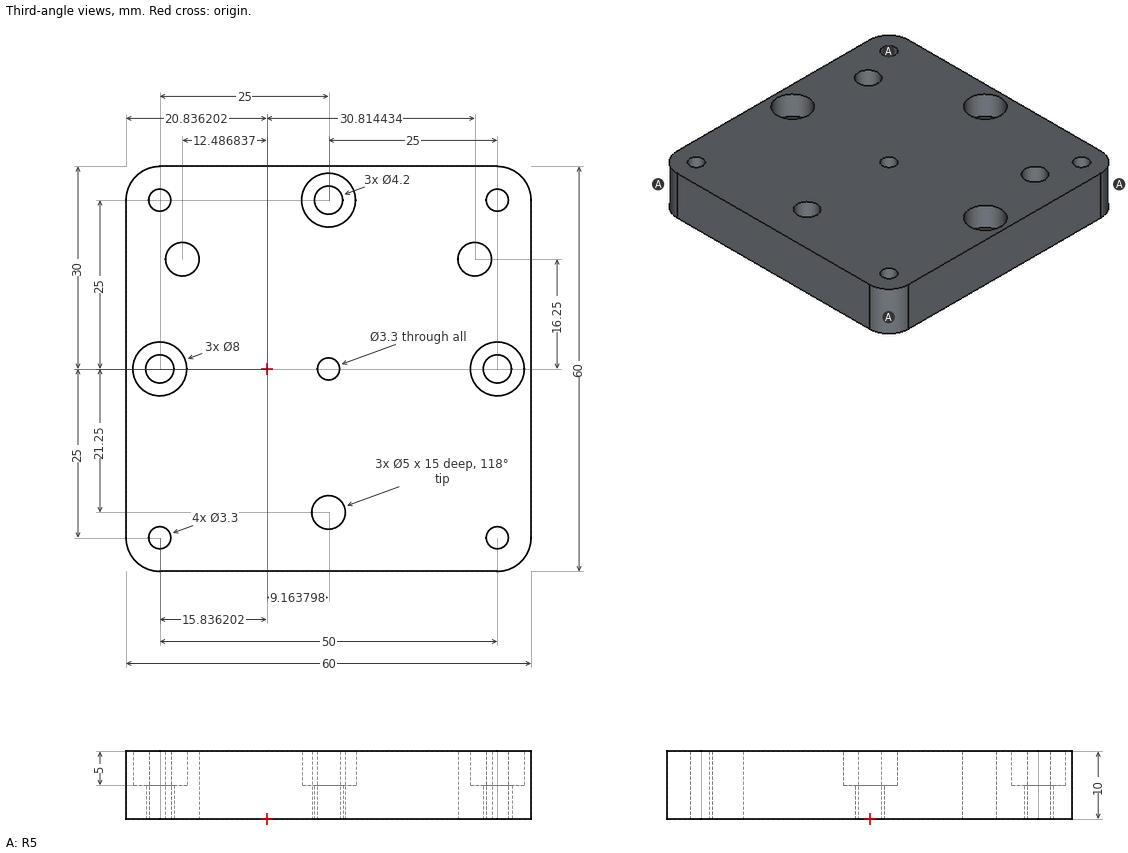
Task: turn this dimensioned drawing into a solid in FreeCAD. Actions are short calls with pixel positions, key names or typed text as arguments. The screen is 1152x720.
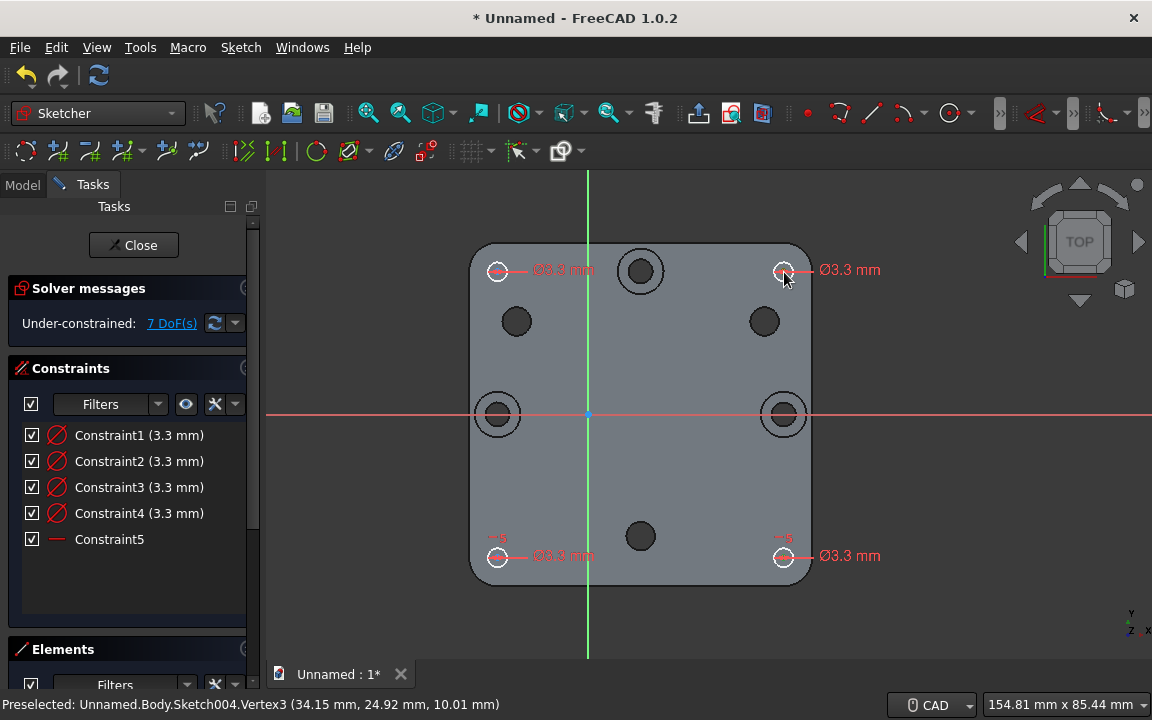
key(v)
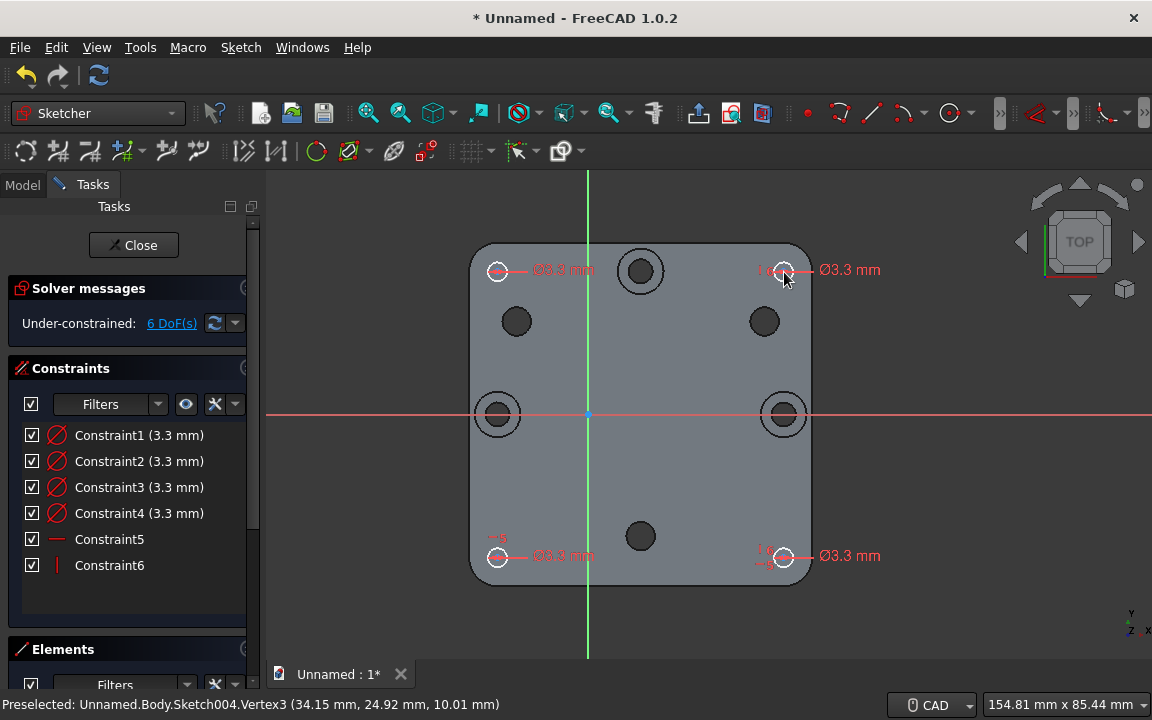
click(498, 558)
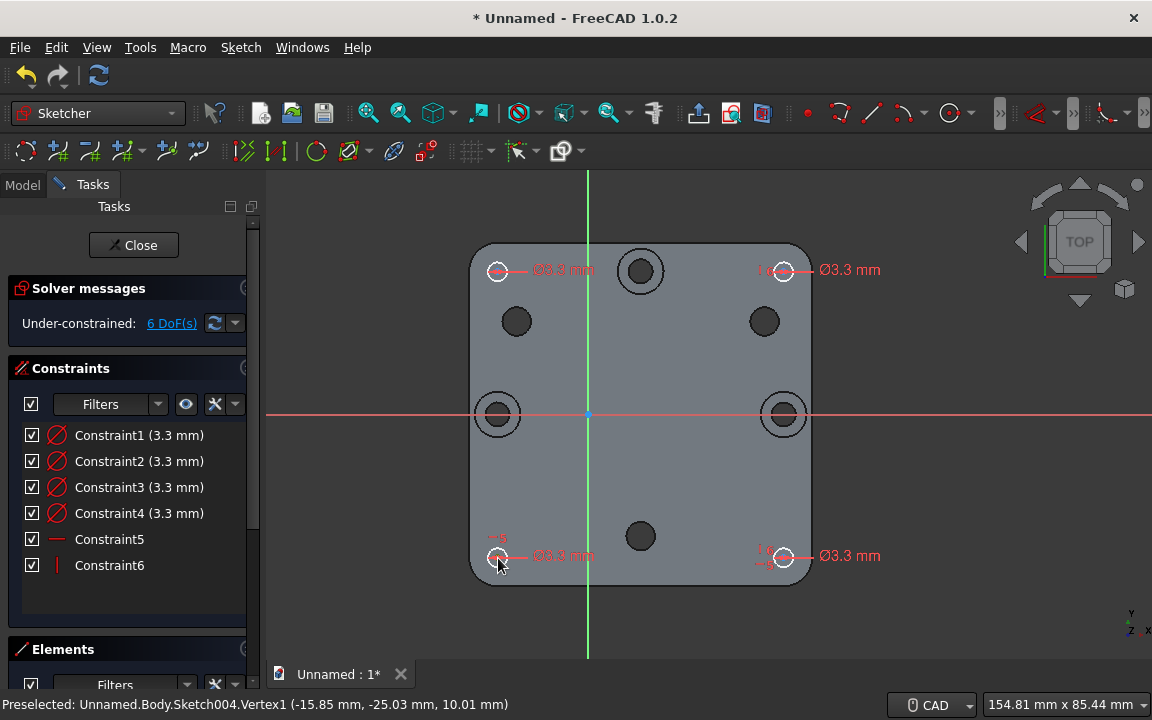
click(497, 272)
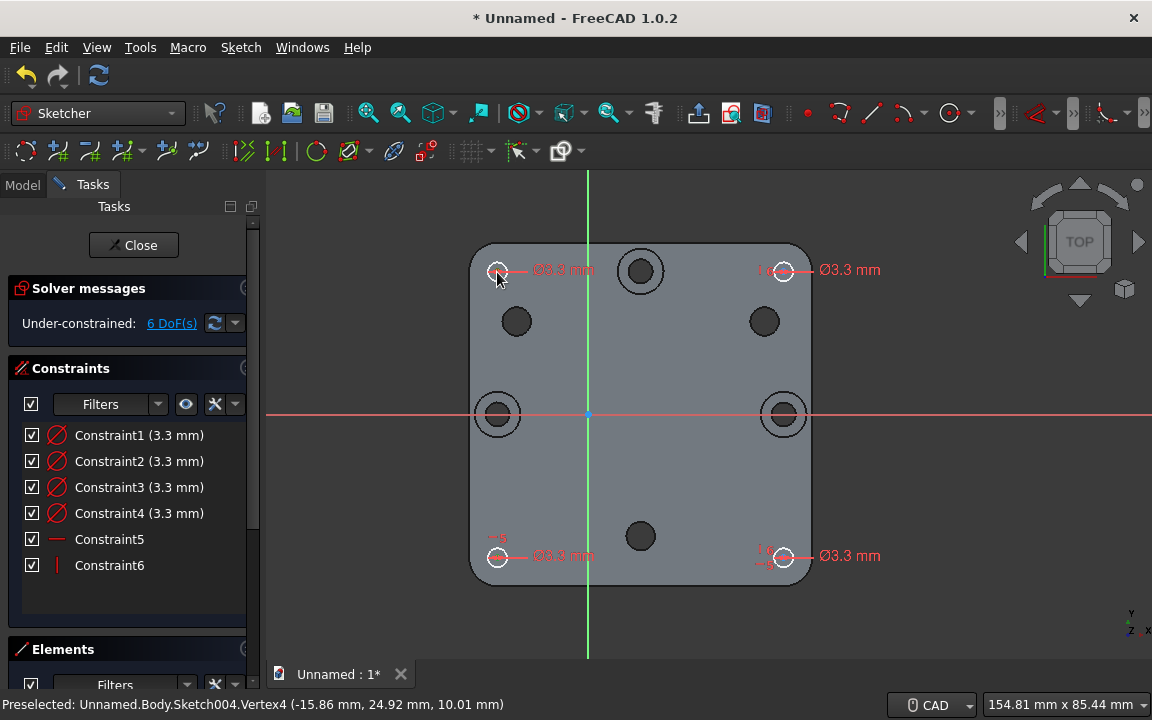
key(v)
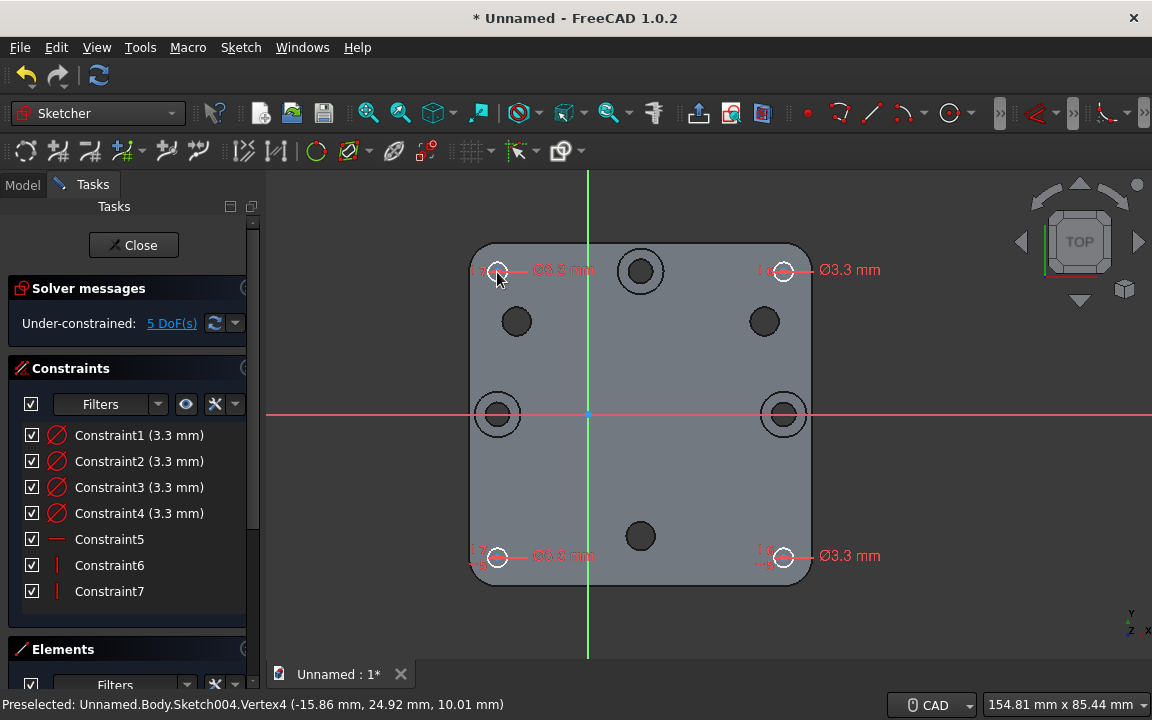
click(784, 272)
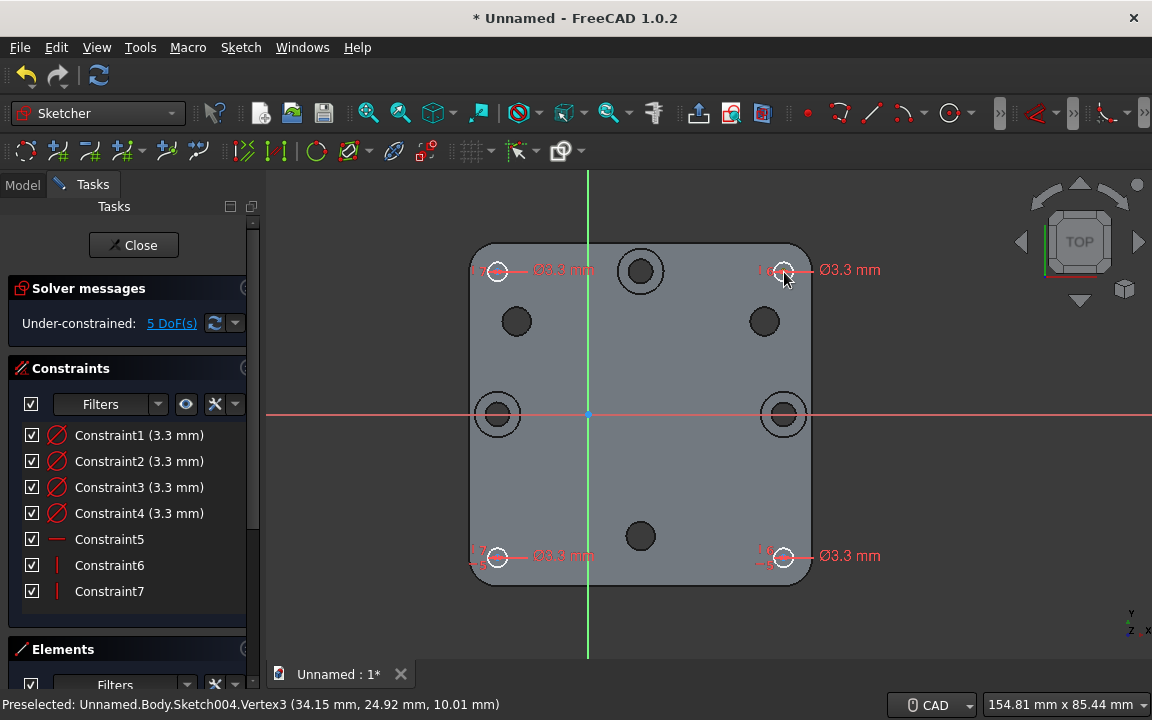
click(498, 272)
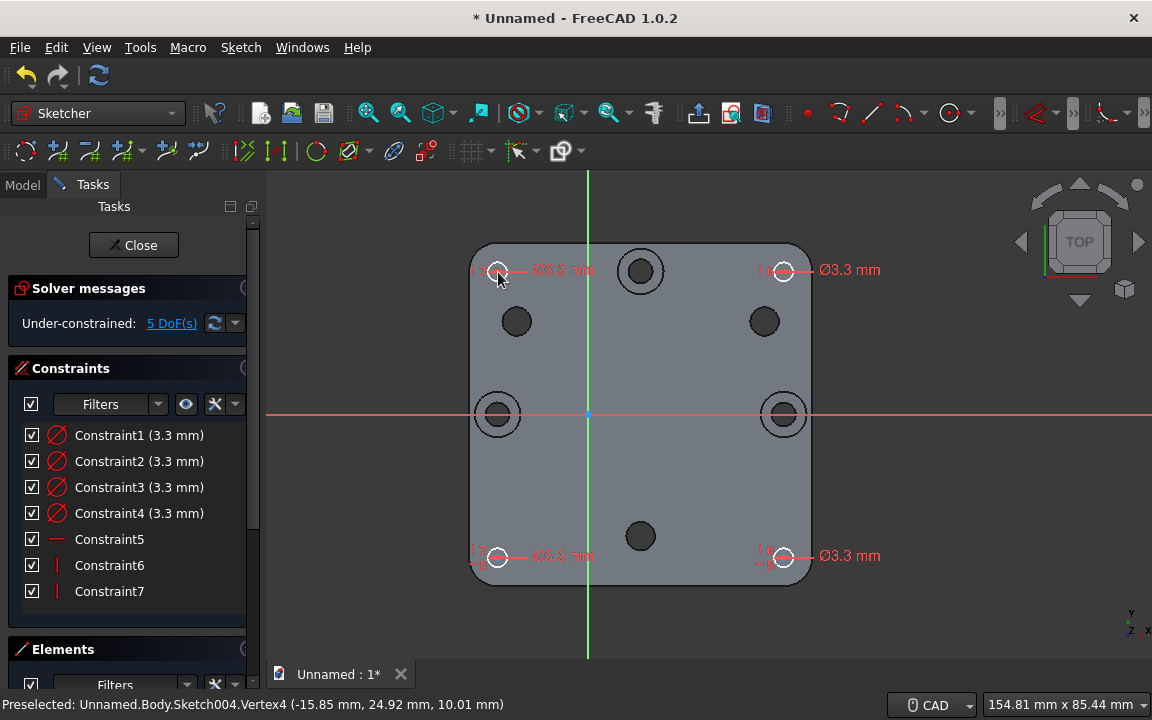
key(h)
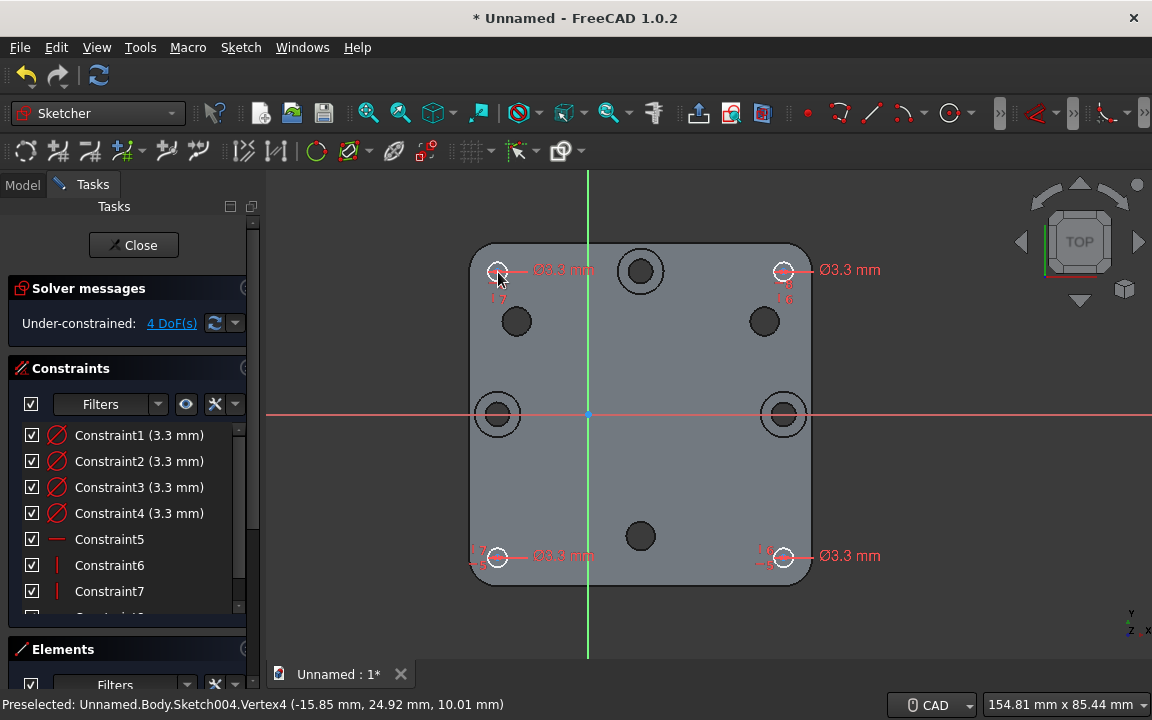
click(1036, 114)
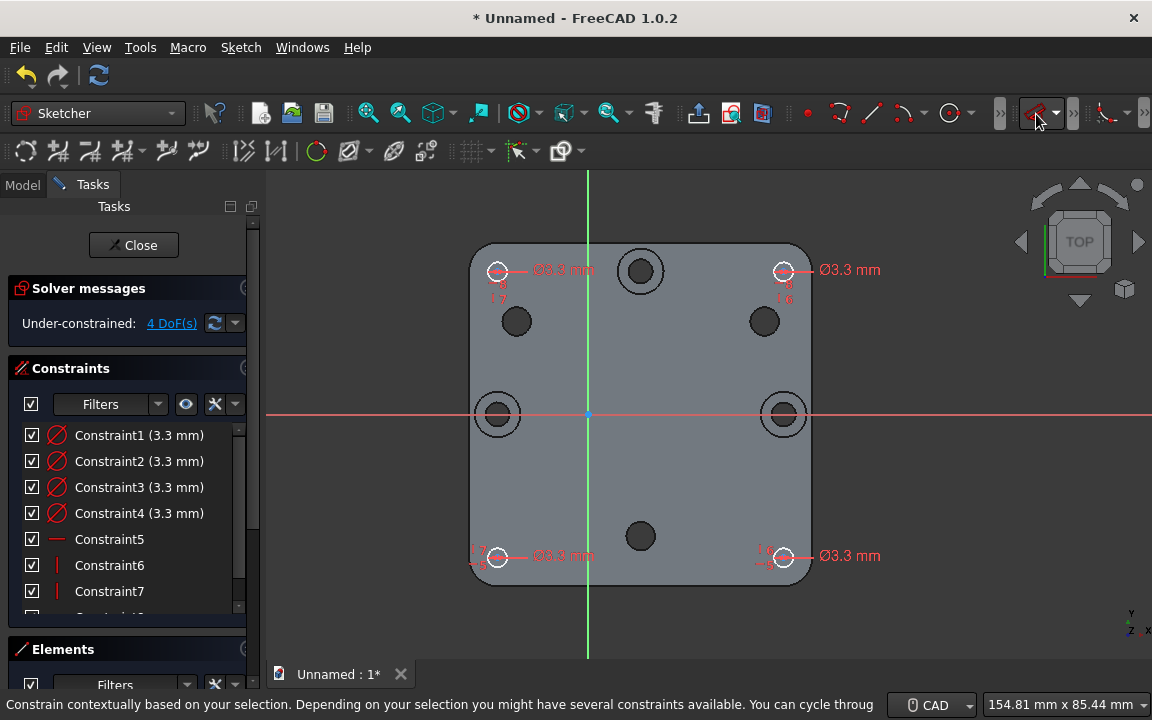
click(498, 558)
click(464, 486)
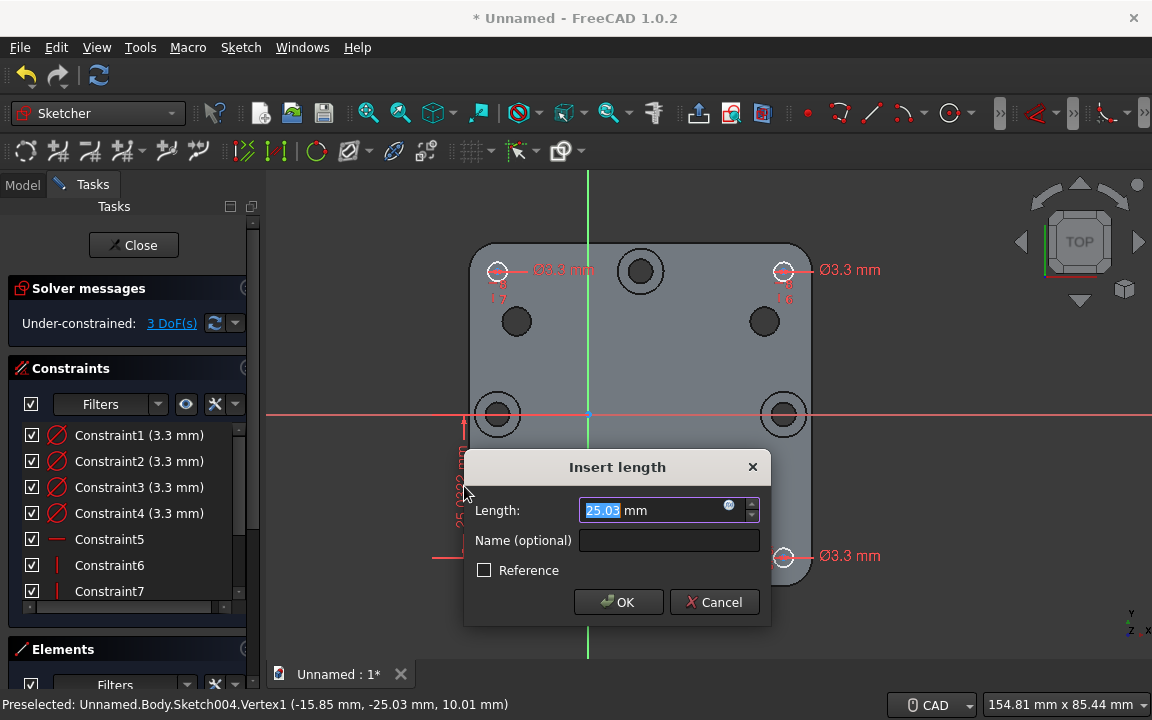
text(25)
key(Return)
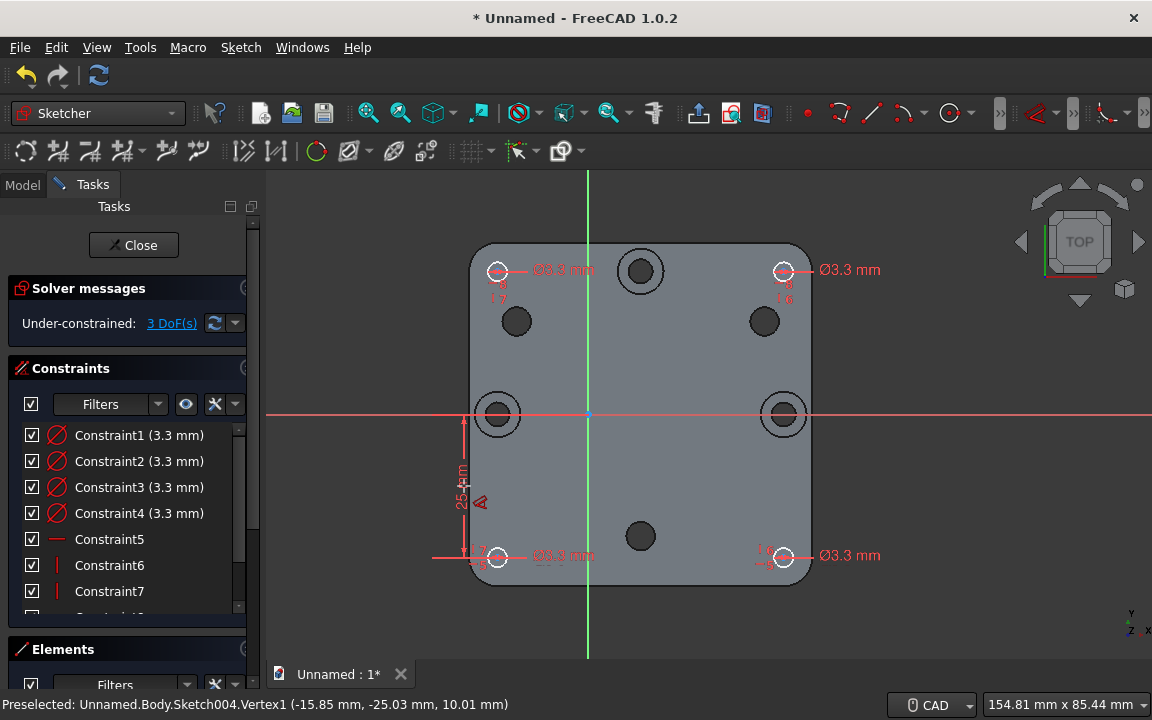
click(784, 272)
click(818, 343)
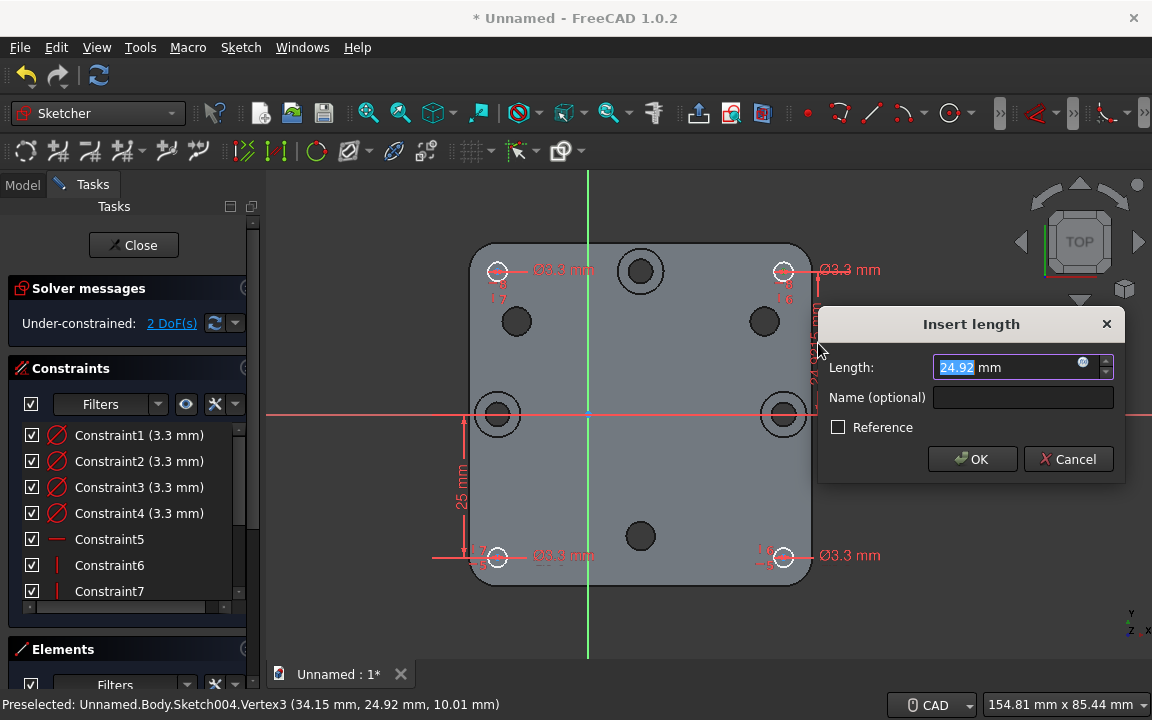
text(25)
key(Return)